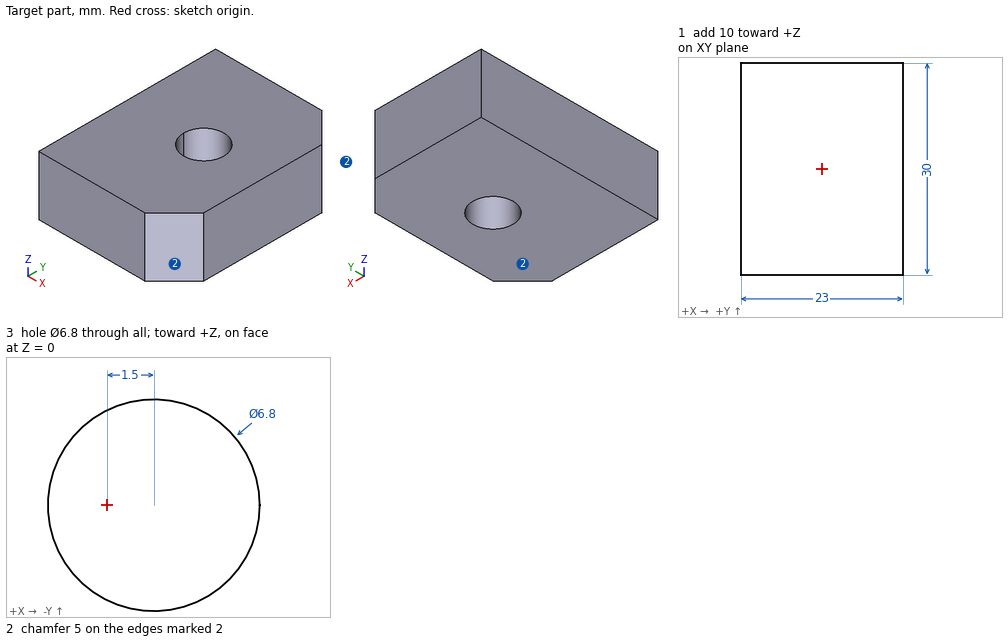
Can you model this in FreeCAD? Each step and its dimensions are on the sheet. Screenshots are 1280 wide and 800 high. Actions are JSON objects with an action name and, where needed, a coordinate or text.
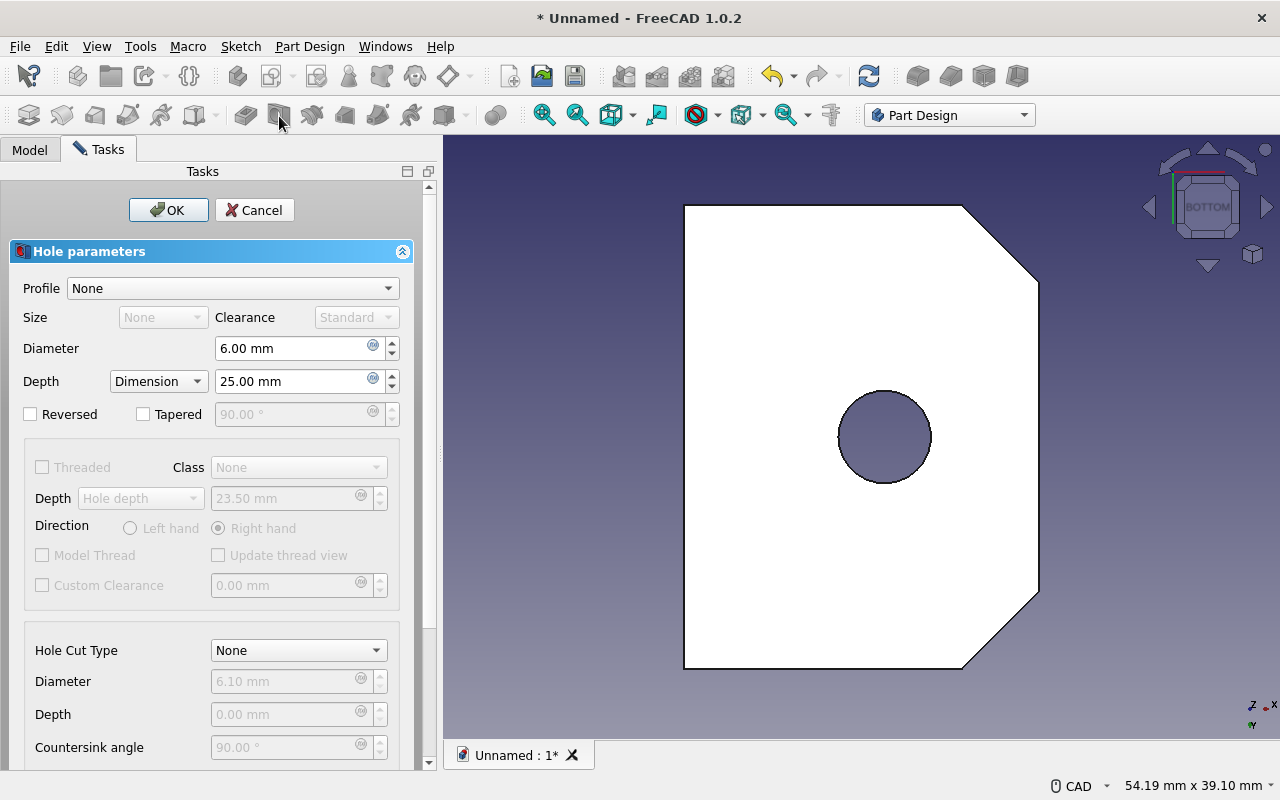
{"action": "triple_click", "coordinate": [300, 348]}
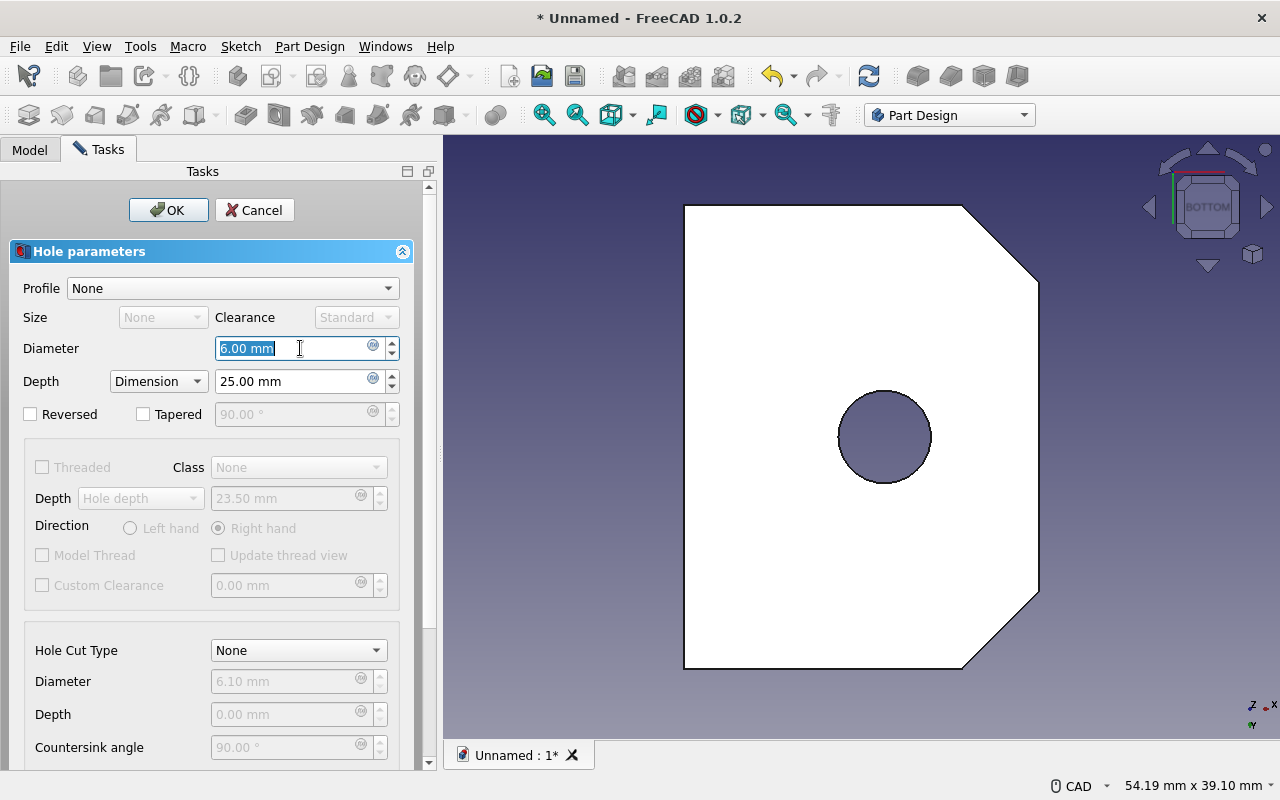
{"action": "type", "text": "6.8"}
{"action": "key", "text": "Tab"}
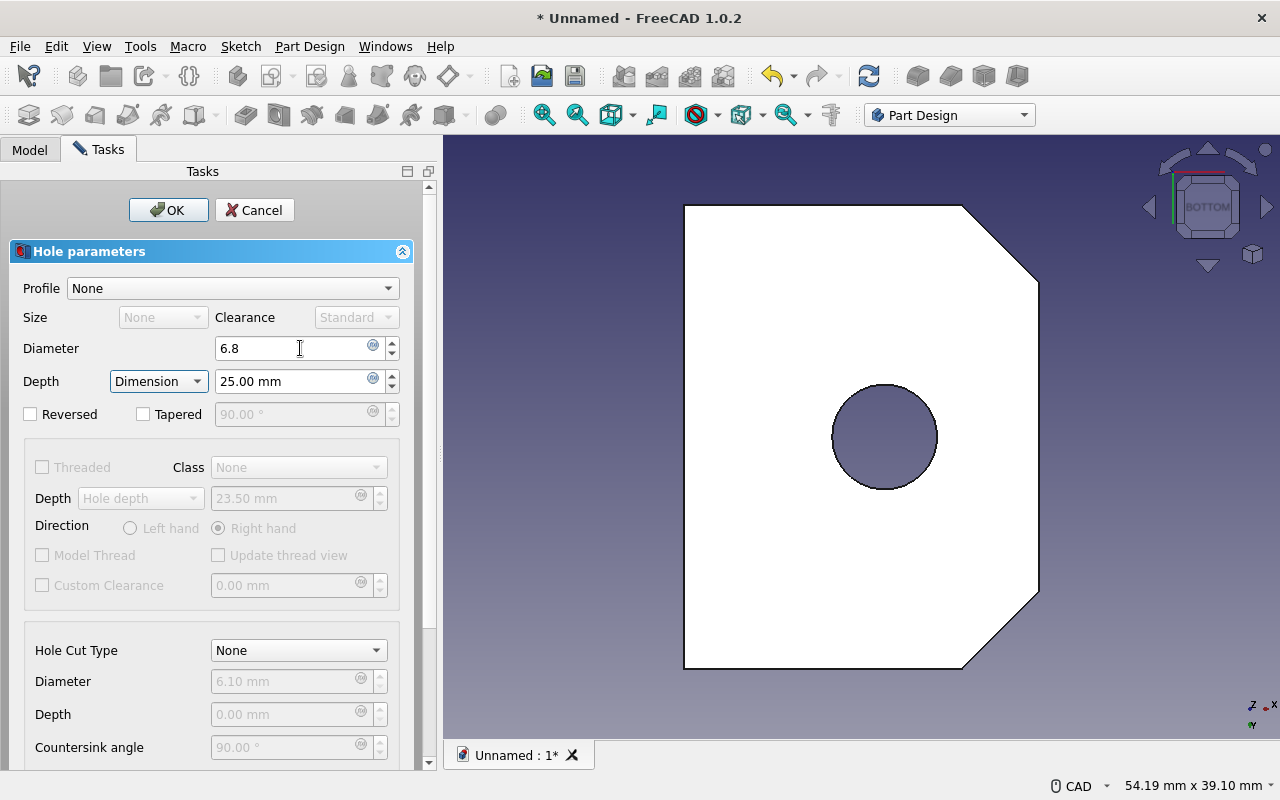
{"action": "left_click", "coordinate": [160, 382]}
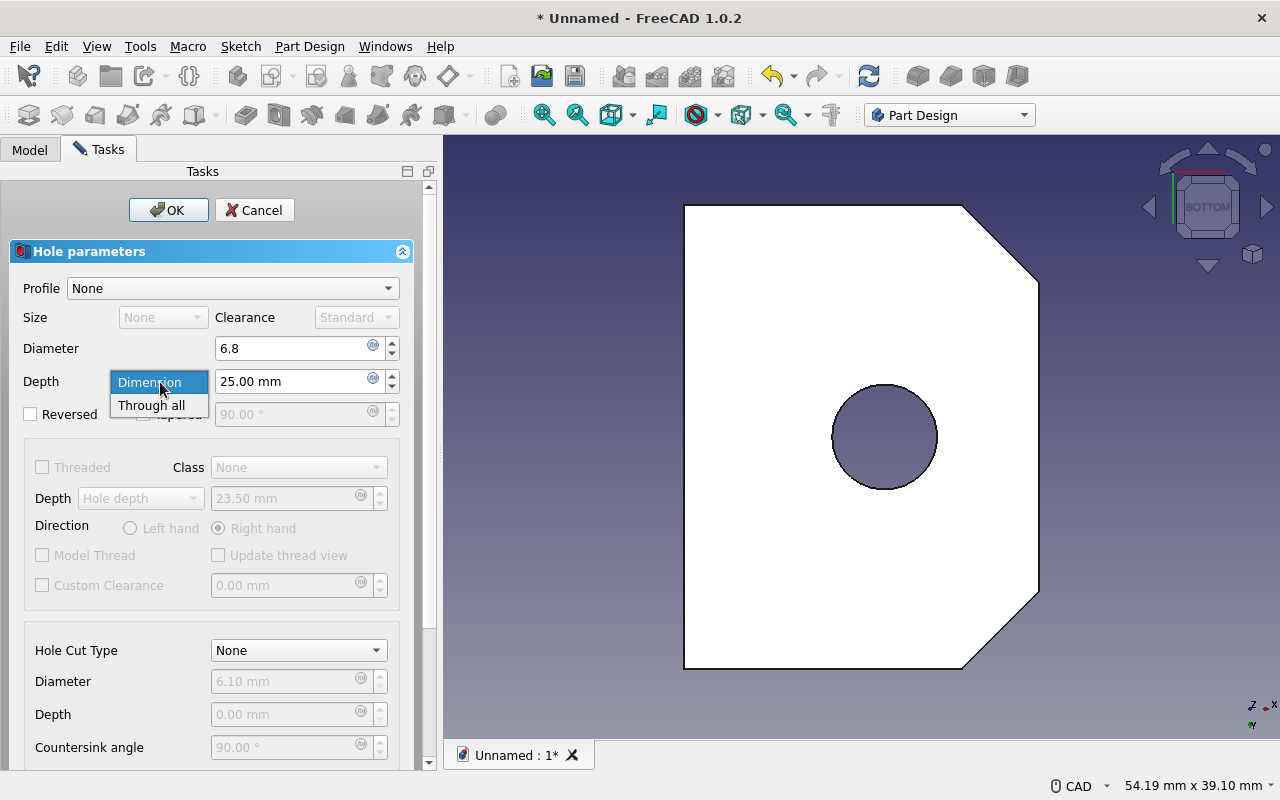
{"action": "left_click", "coordinate": [158, 406]}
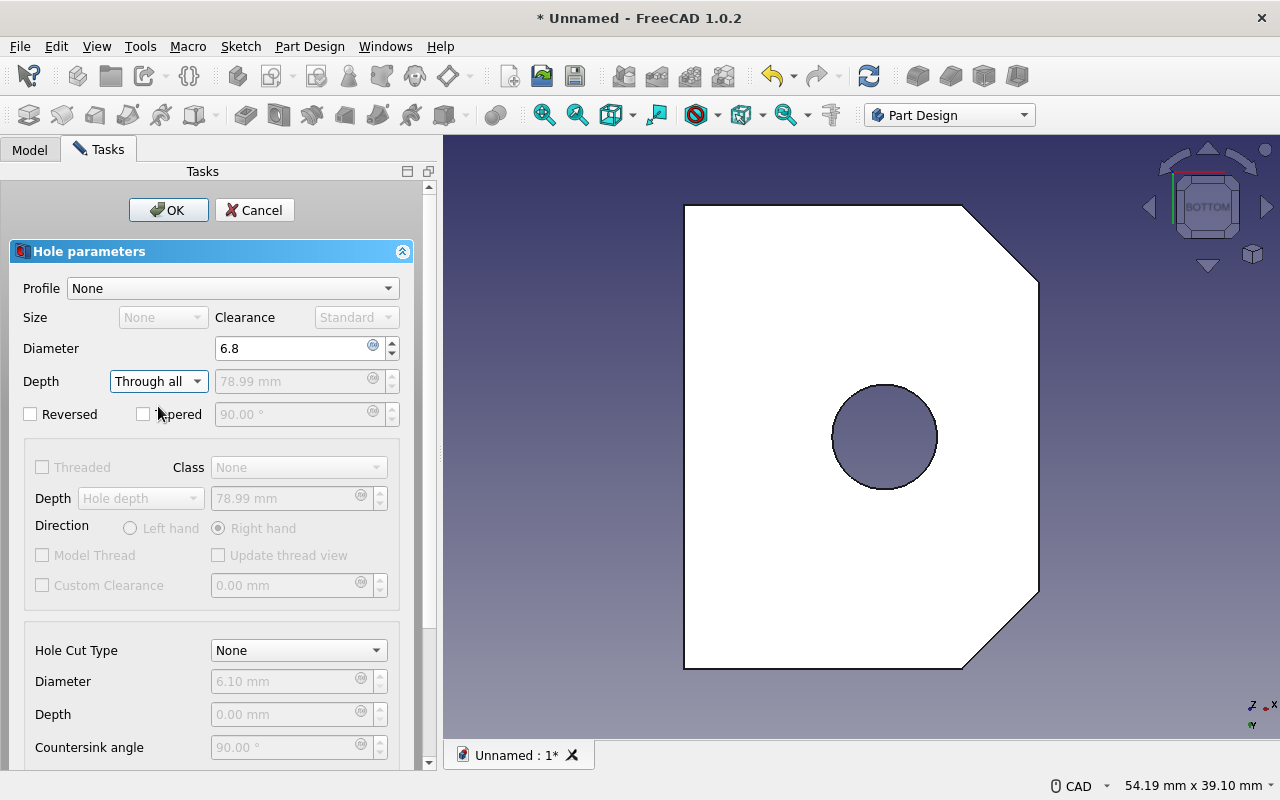
{"action": "left_click", "coordinate": [169, 210]}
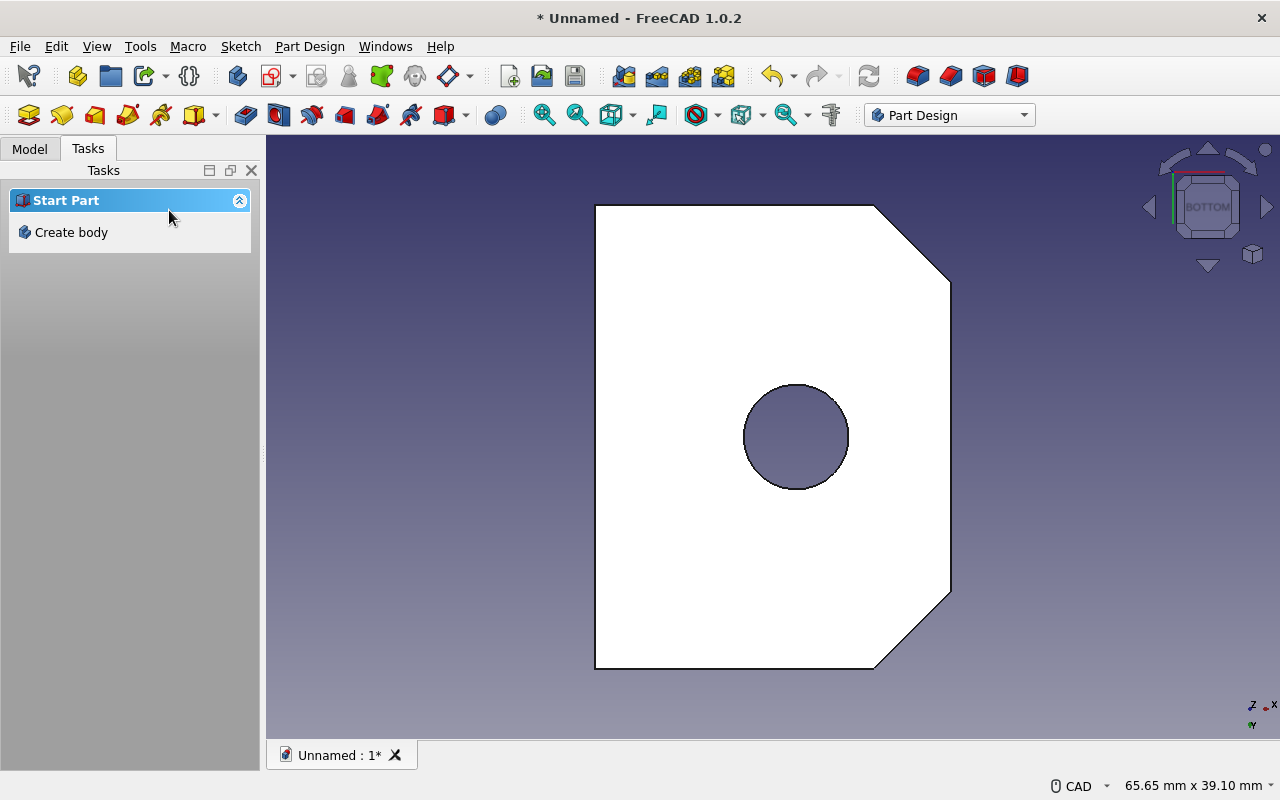
{"action": "key", "text": "0"}